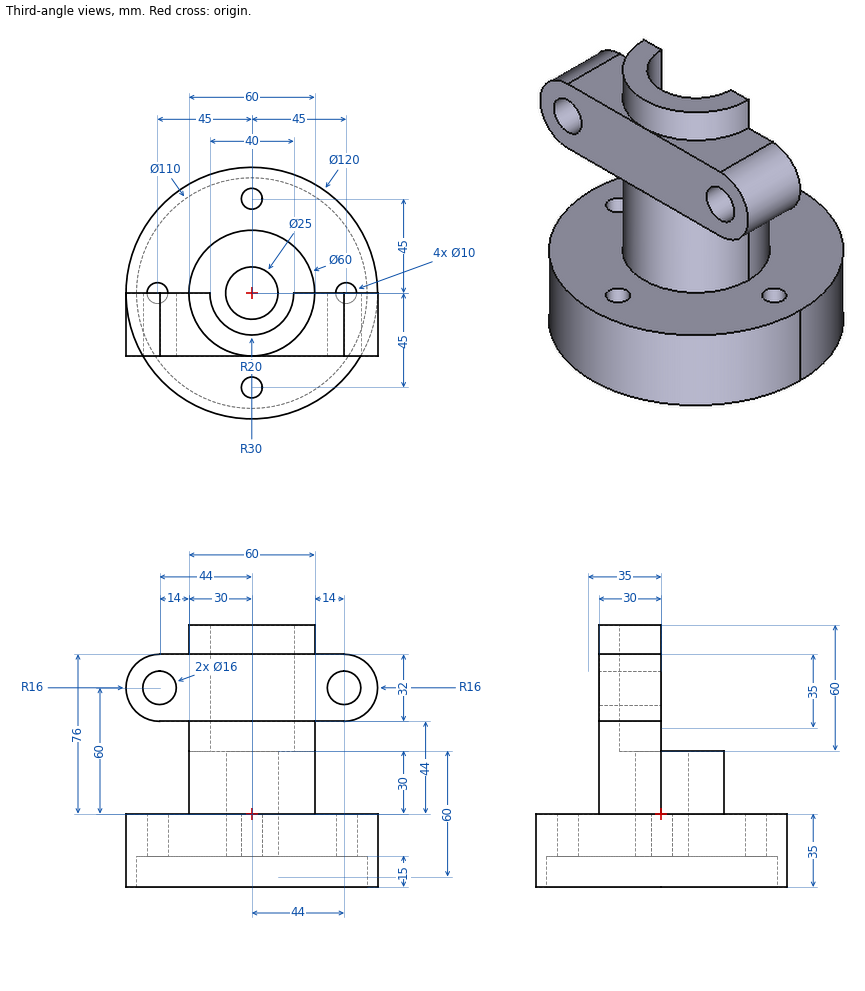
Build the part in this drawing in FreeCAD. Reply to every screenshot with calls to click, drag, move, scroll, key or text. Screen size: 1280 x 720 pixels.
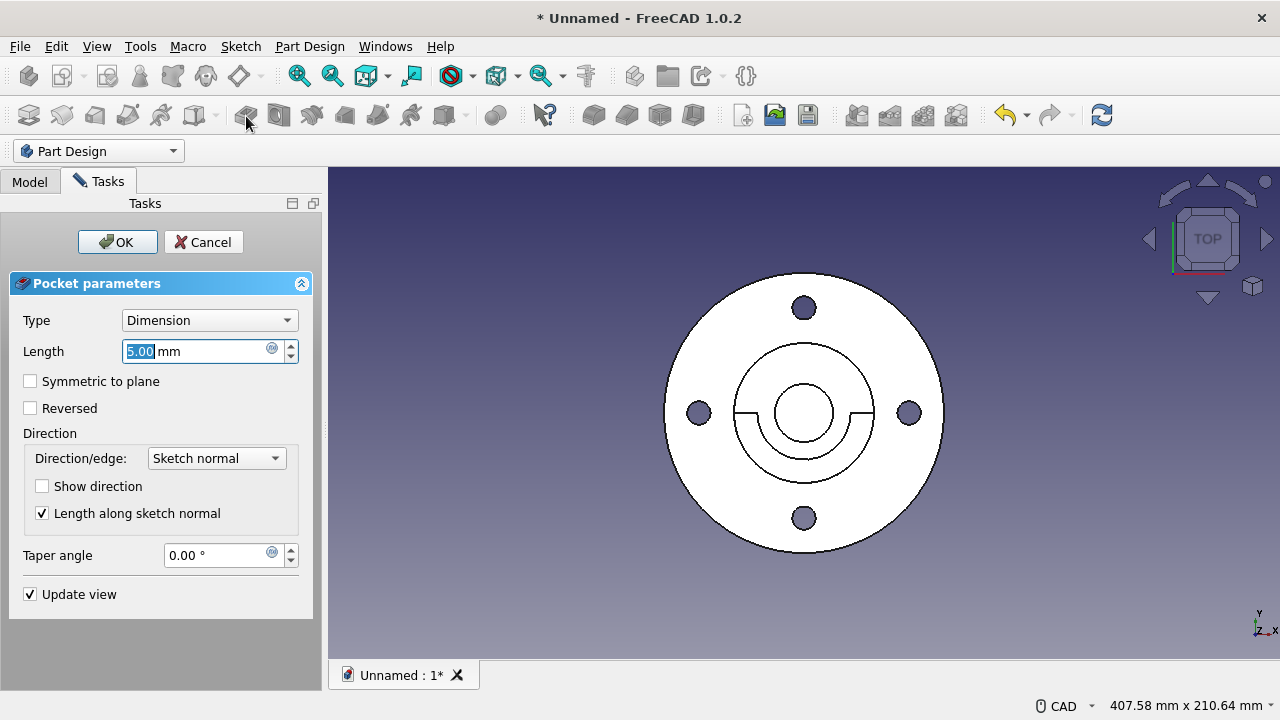
text(60)
key(Tab)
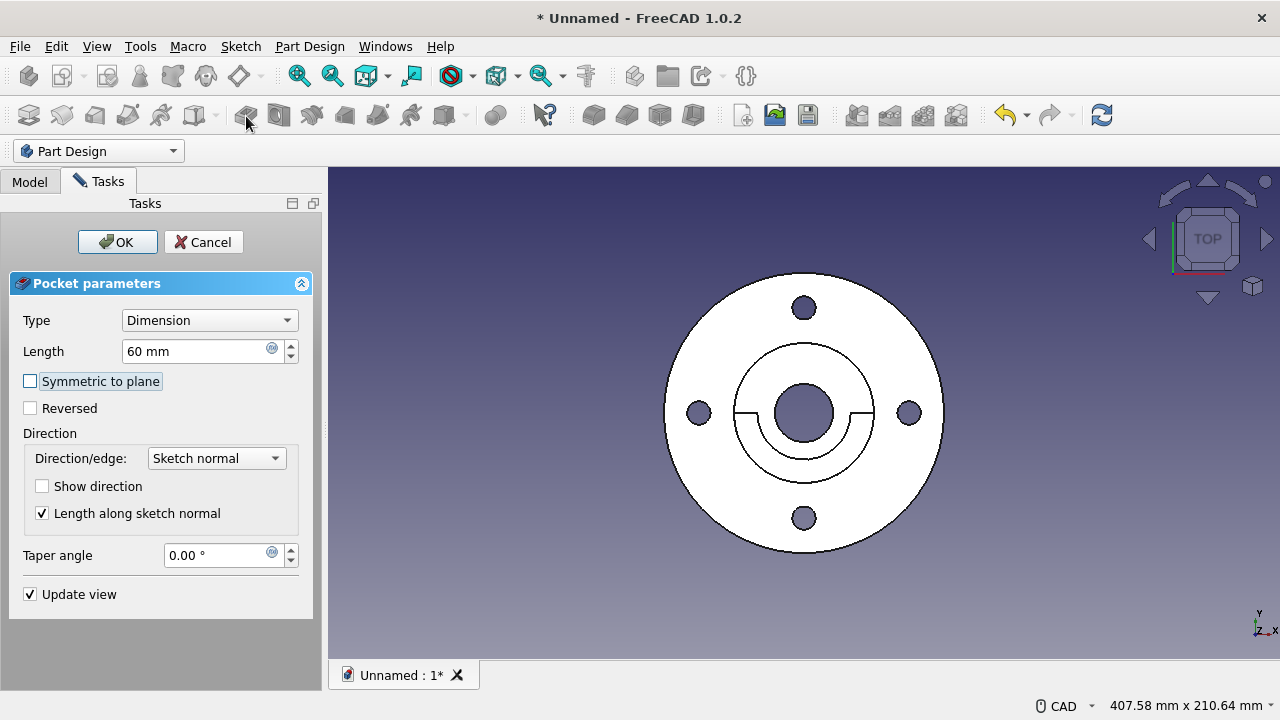
click(118, 242)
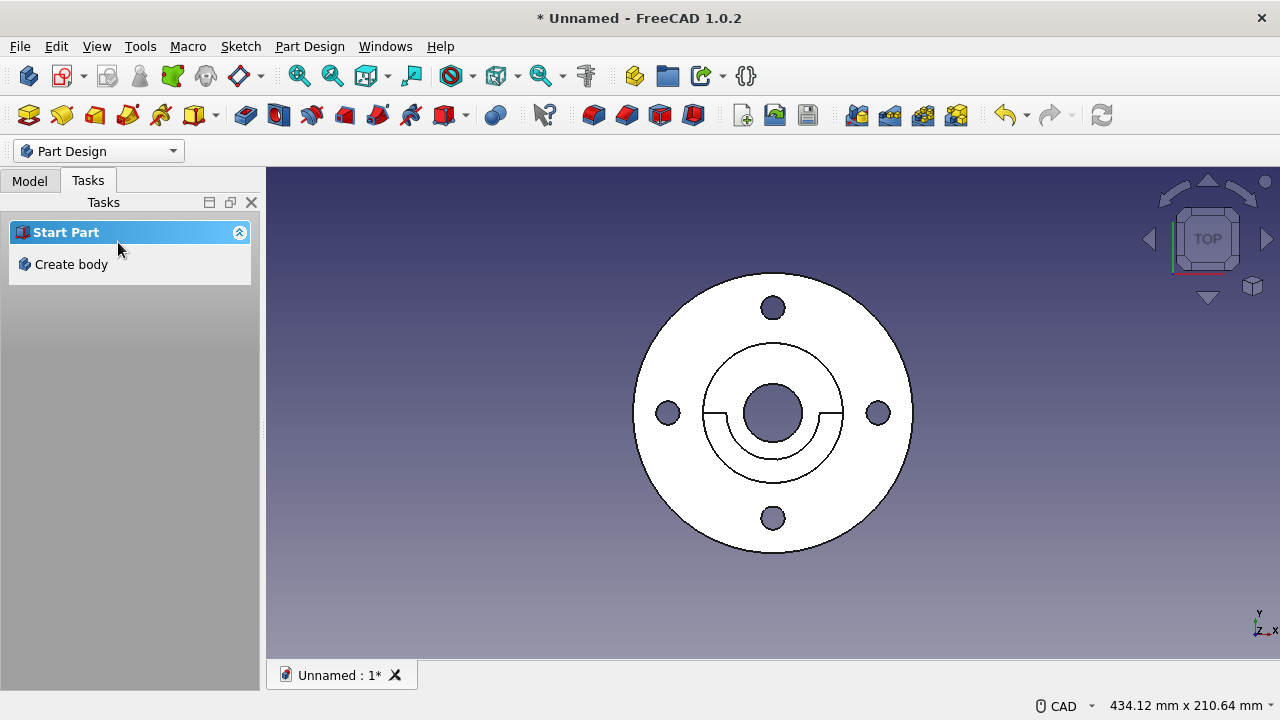
click(29, 76)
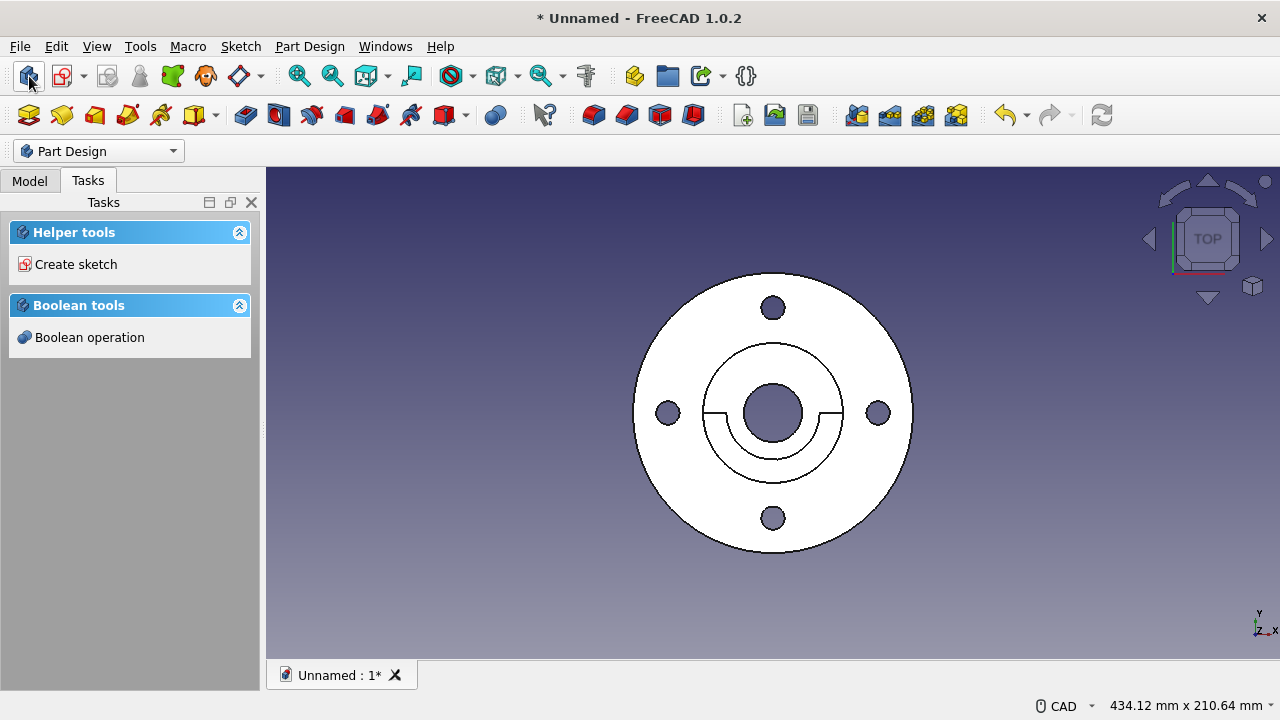
click(306, 619)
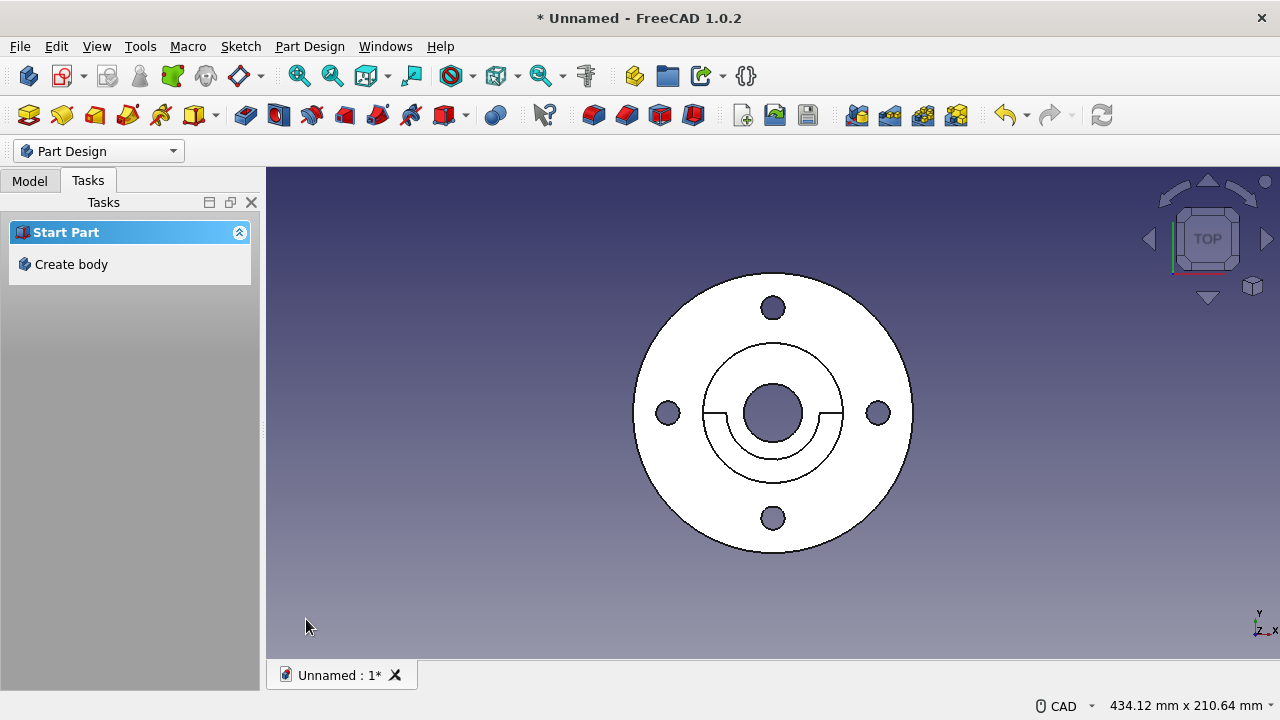
click(62, 76)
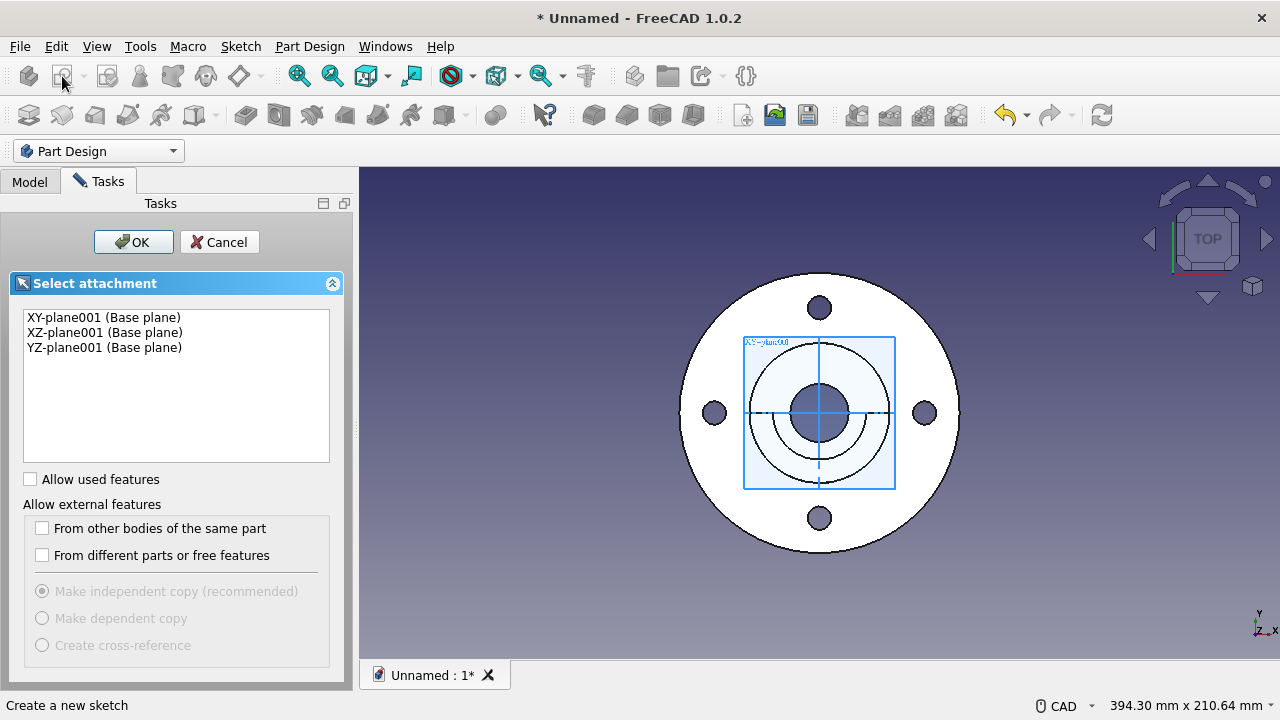
click(84, 332)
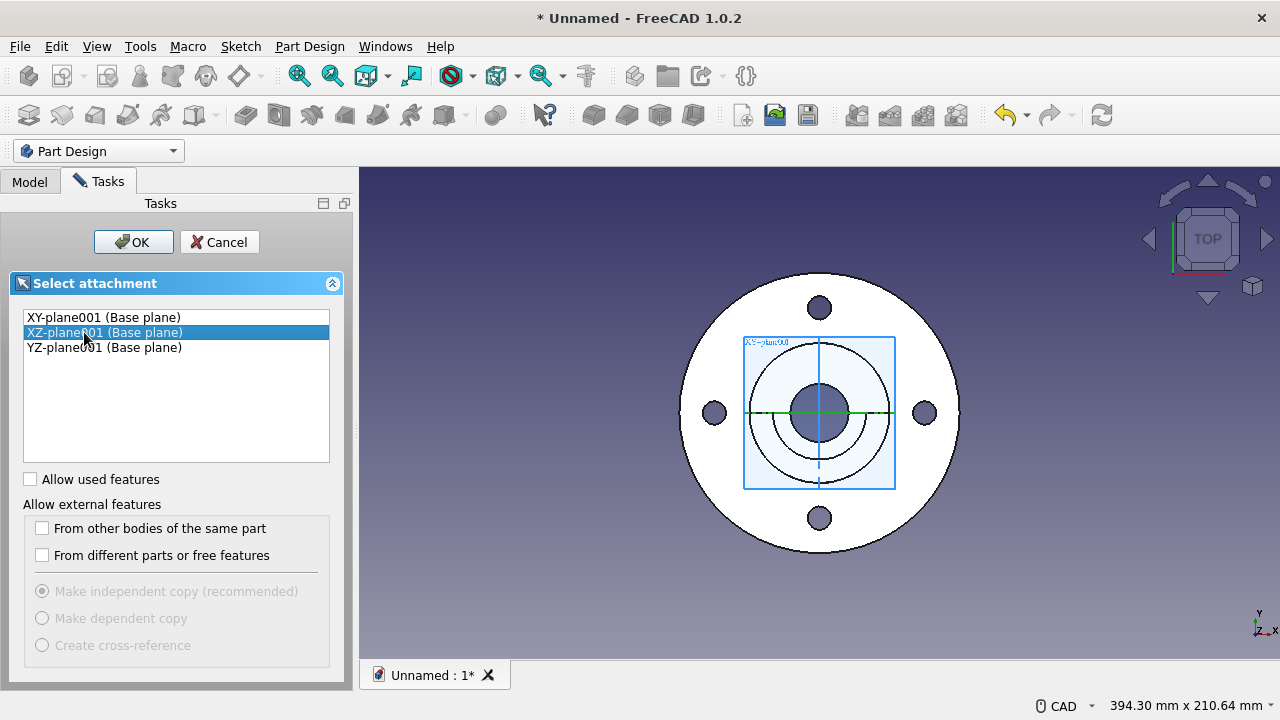
click(134, 242)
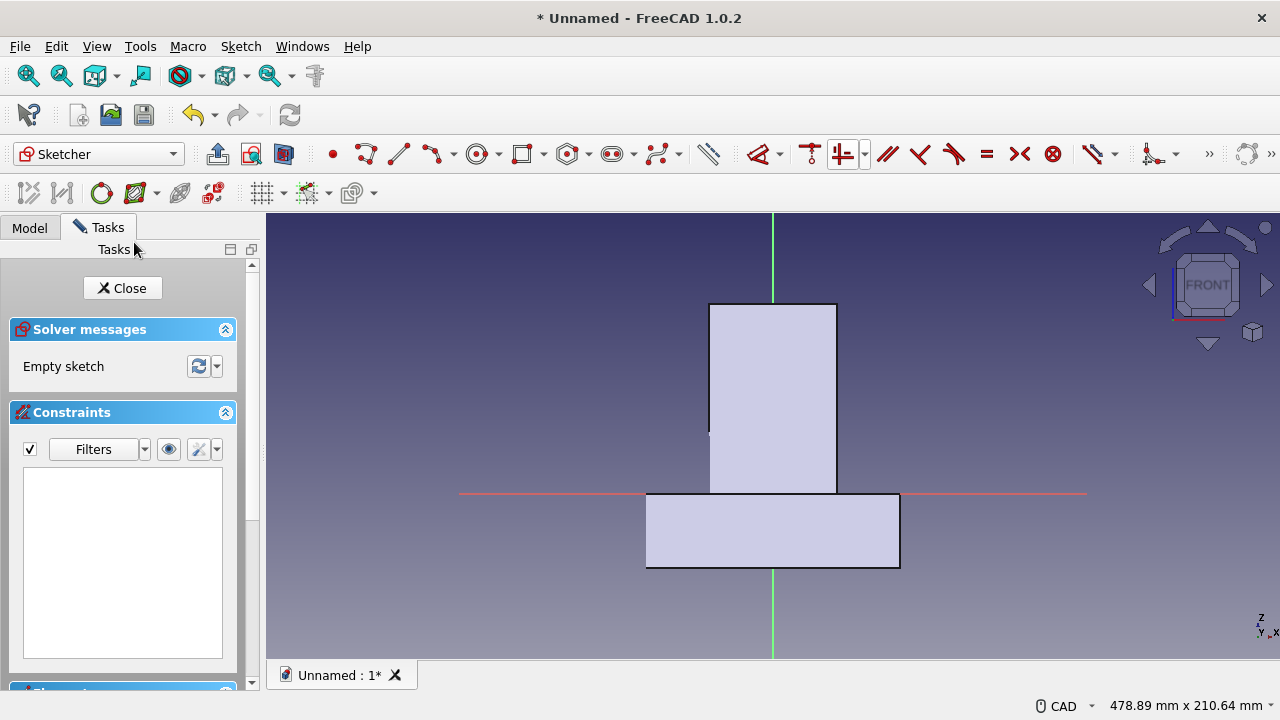
scroll(716, 387, up, 3)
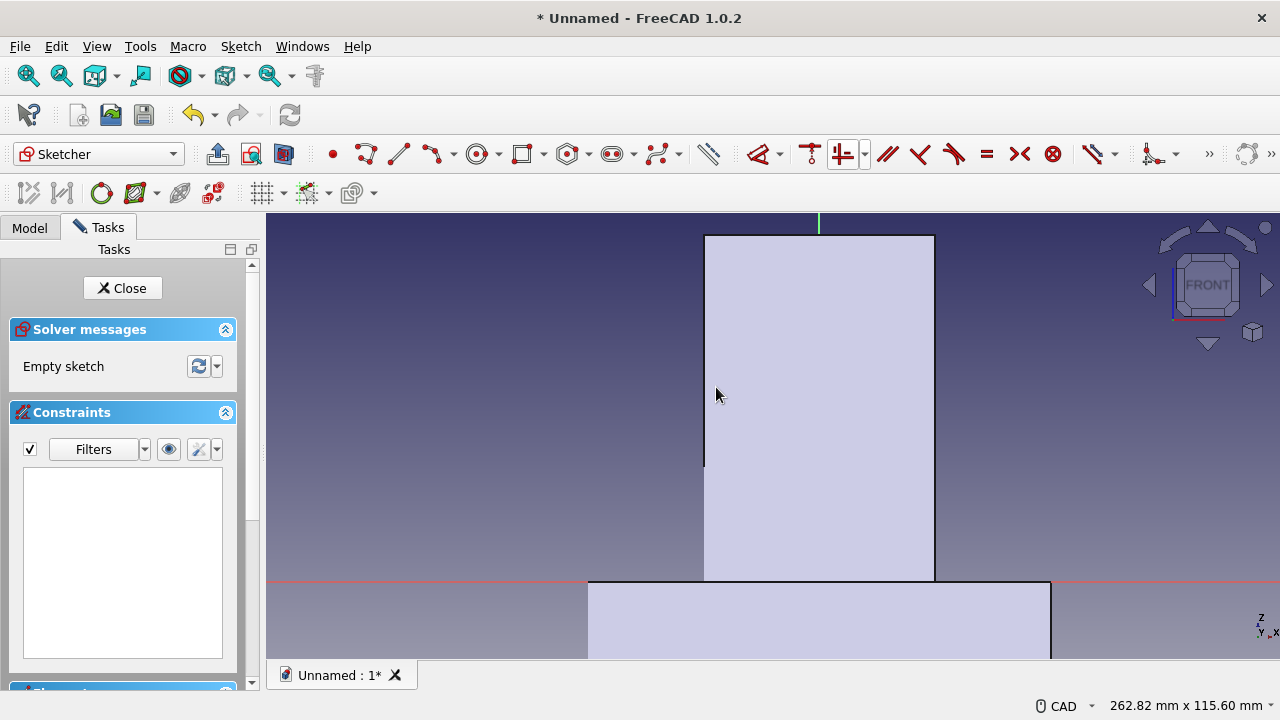
click(366, 154)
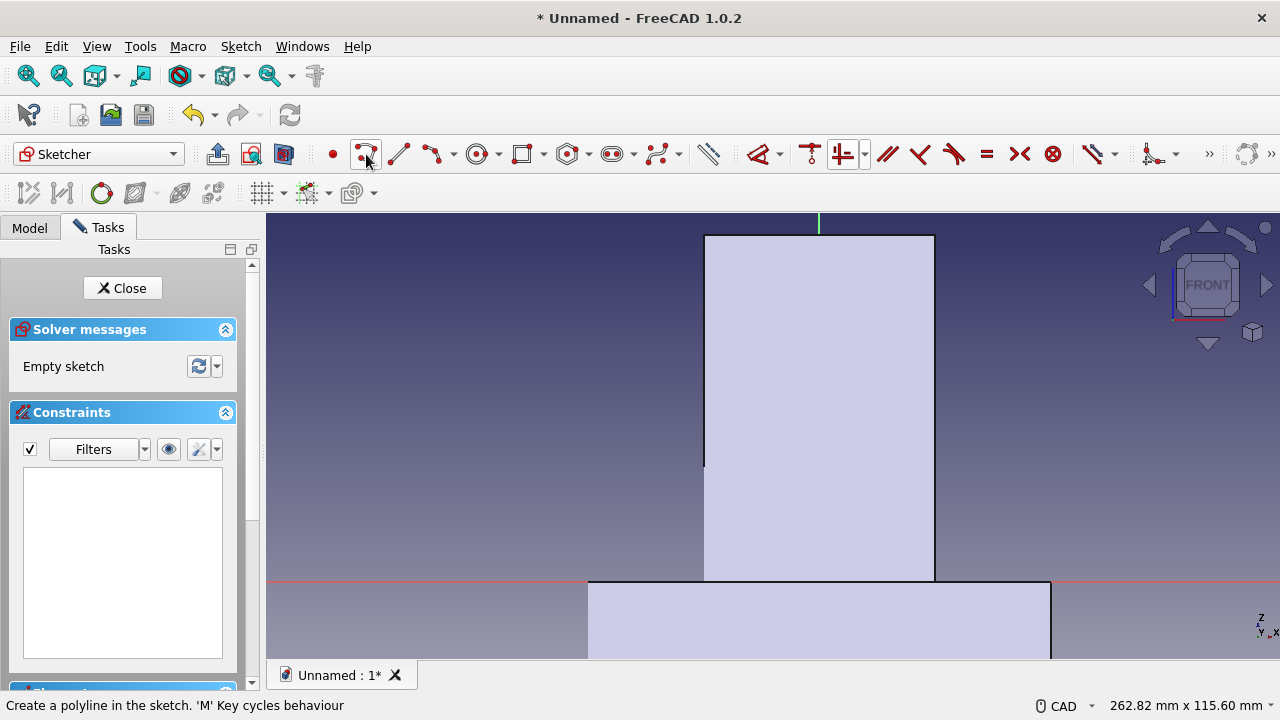
click(650, 289)
click(704, 289)
click(704, 412)
click(650, 412)
right_click(650, 412)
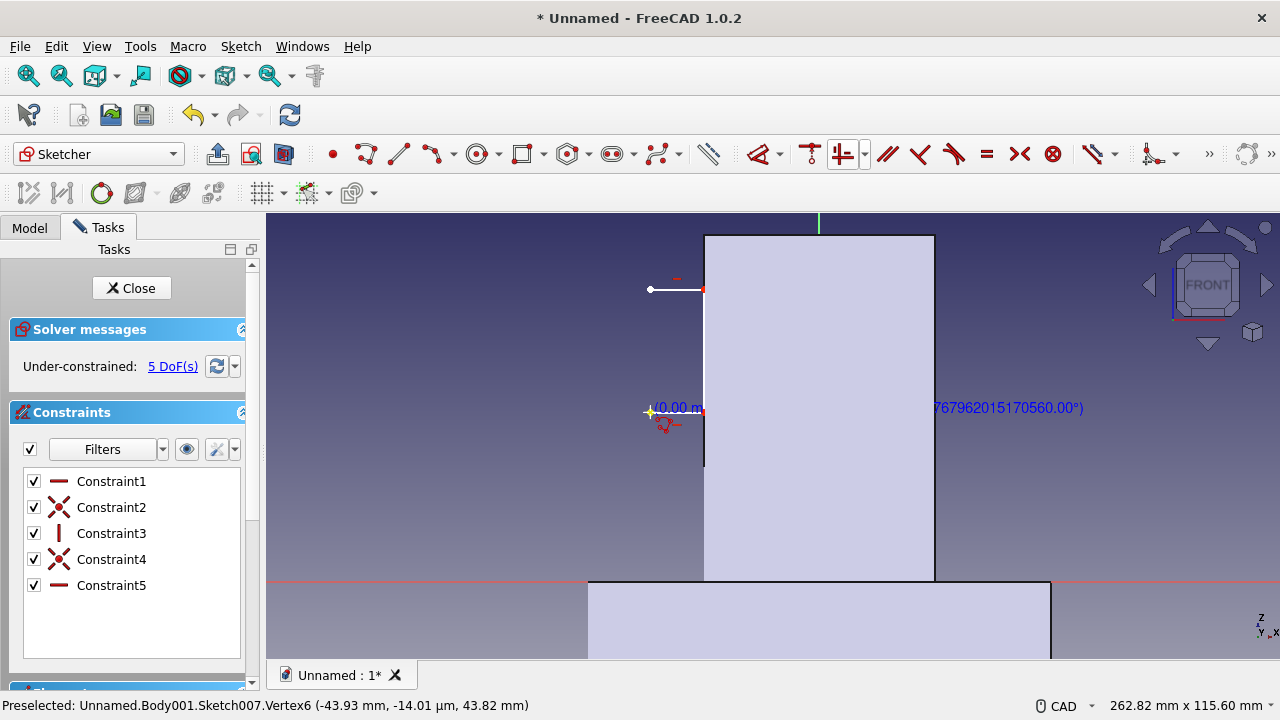
click(432, 154)